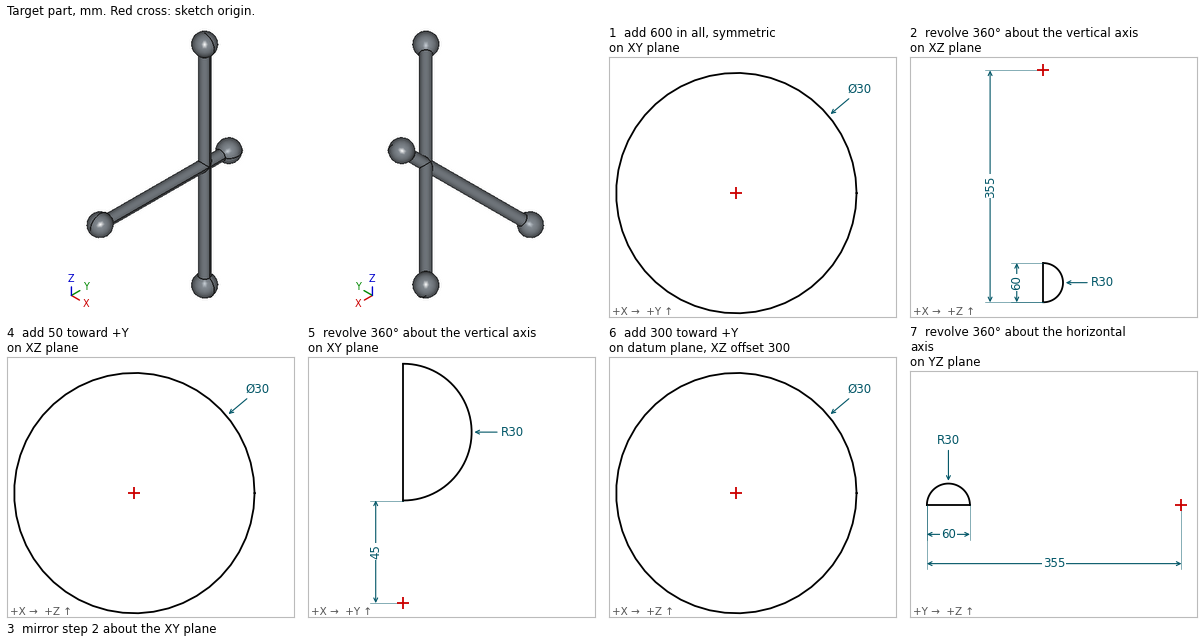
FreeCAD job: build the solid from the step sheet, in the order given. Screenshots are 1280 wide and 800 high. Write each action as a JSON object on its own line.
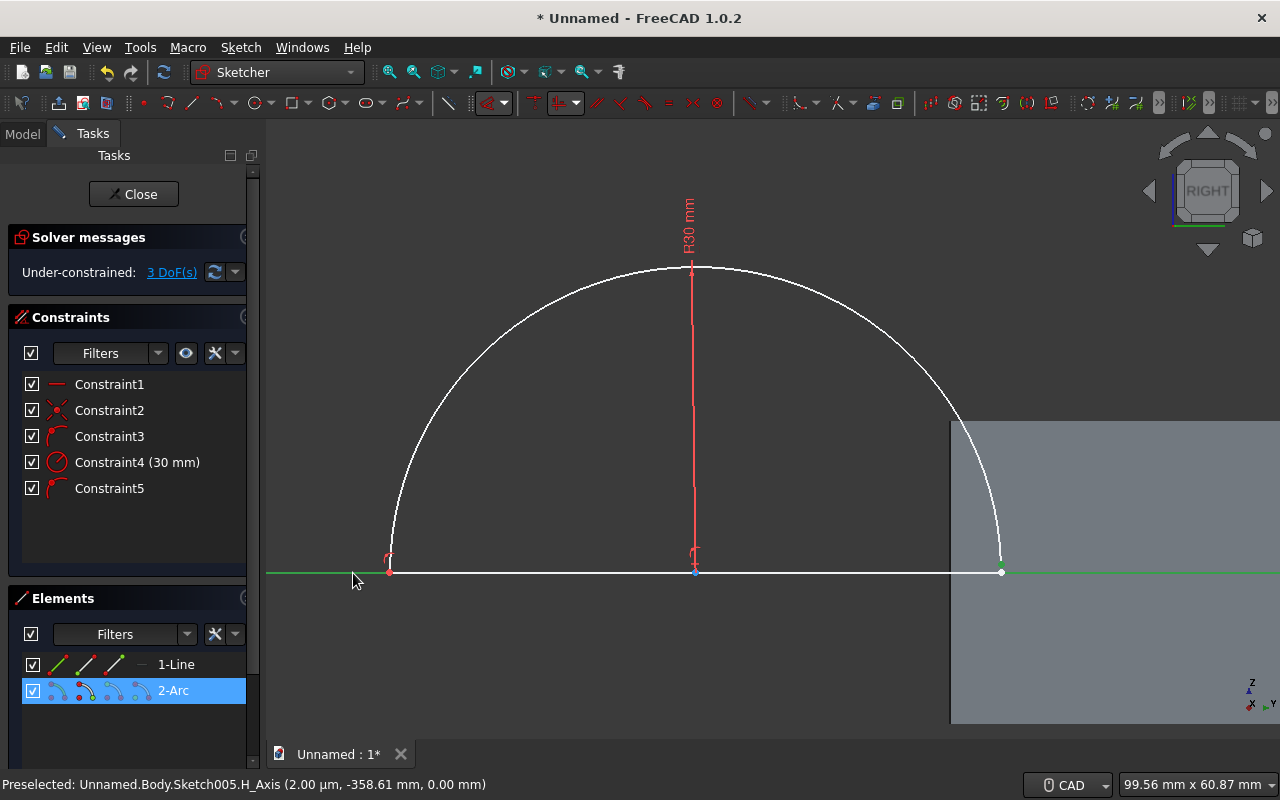
{"action": "left_click", "coordinate": [534, 104]}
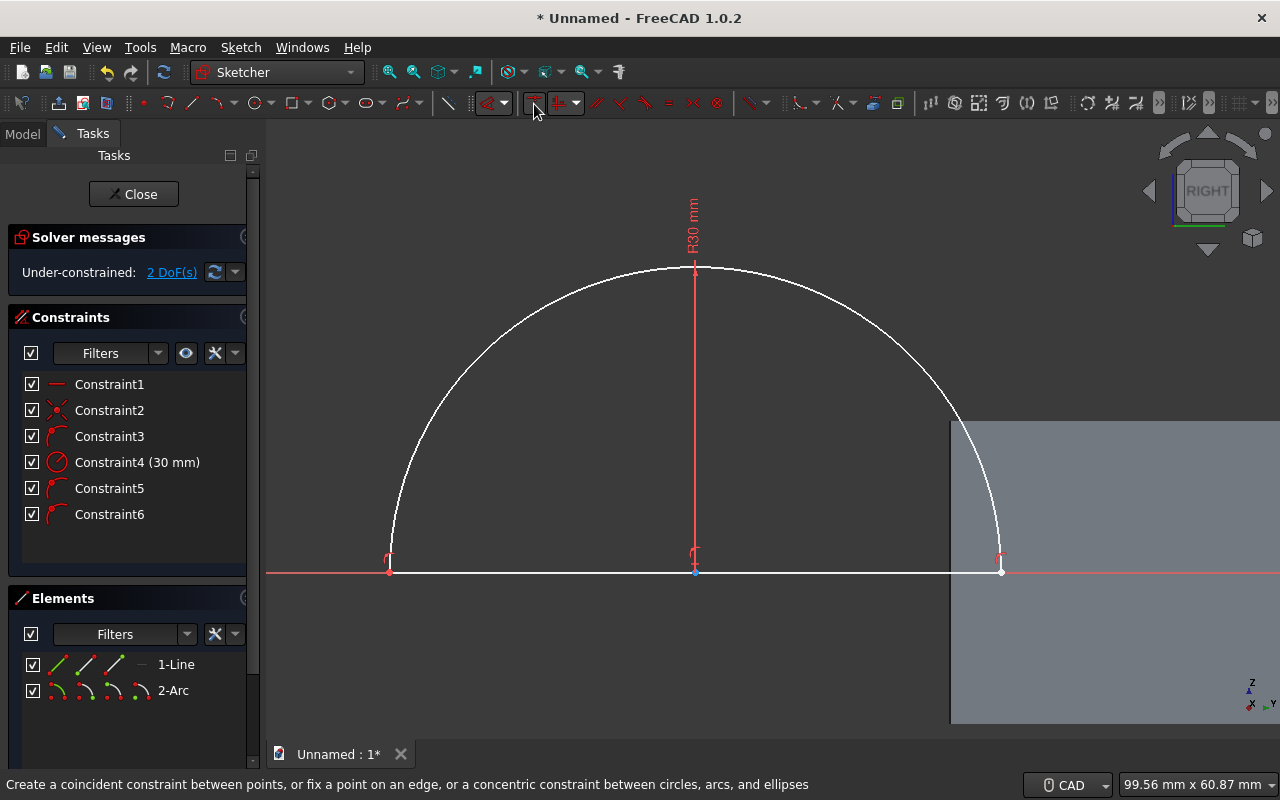
{"action": "left_click", "coordinate": [573, 573]}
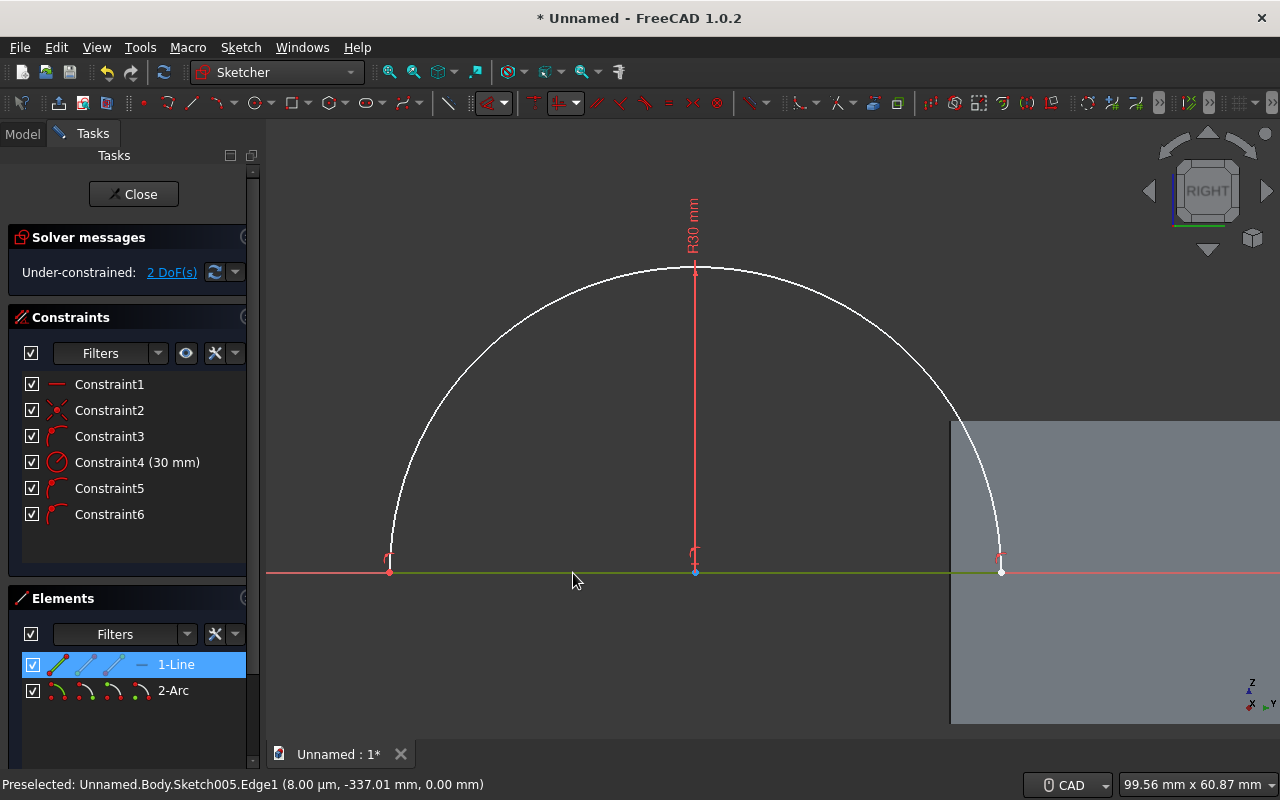
{"action": "key", "text": "l"}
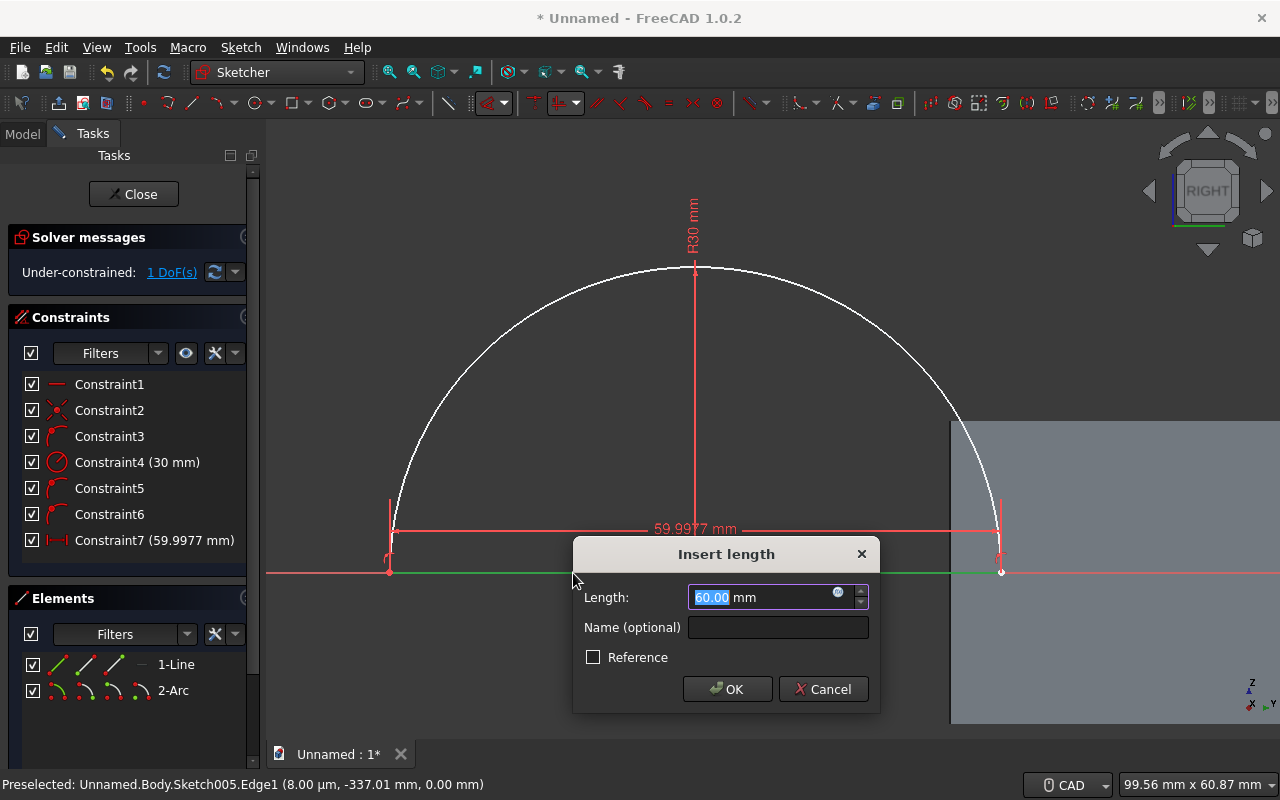
{"action": "type", "text": "60"}
{"action": "key", "text": "Return"}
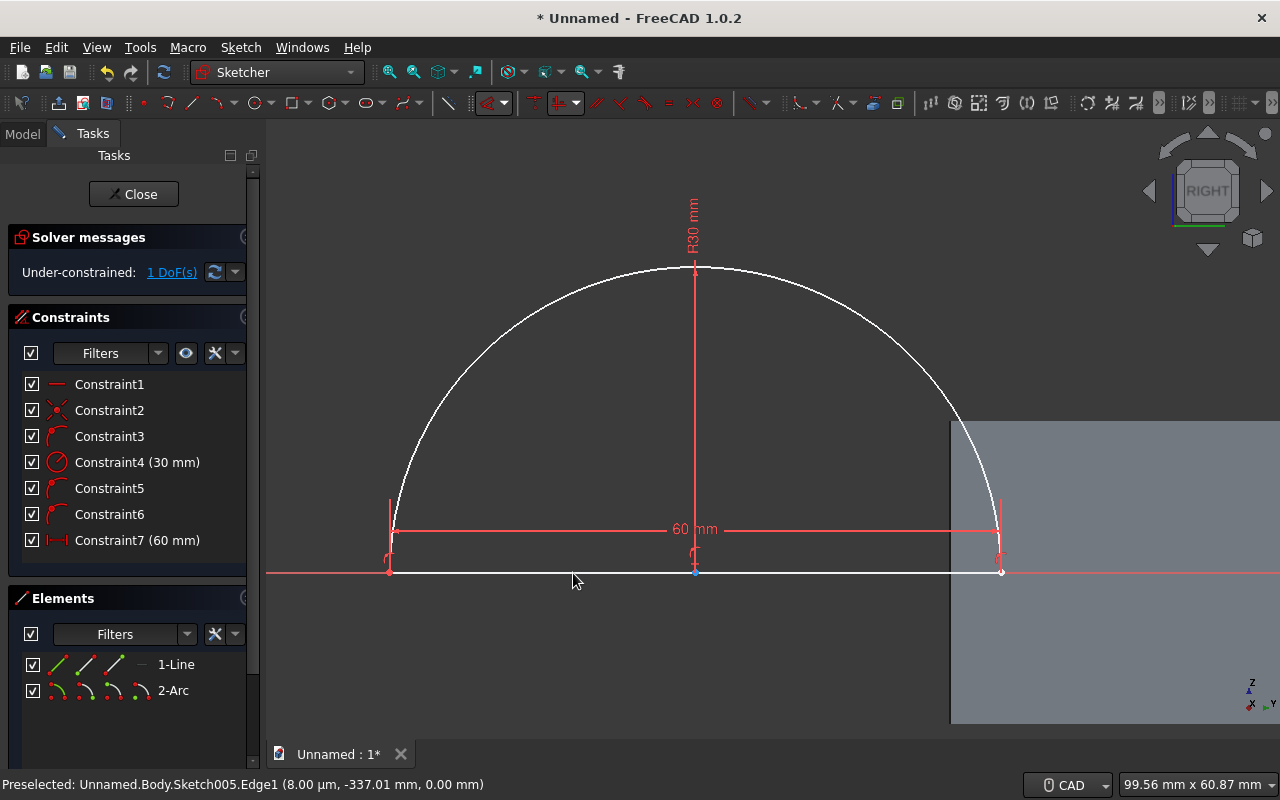
{"action": "left_click", "coordinate": [390, 573]}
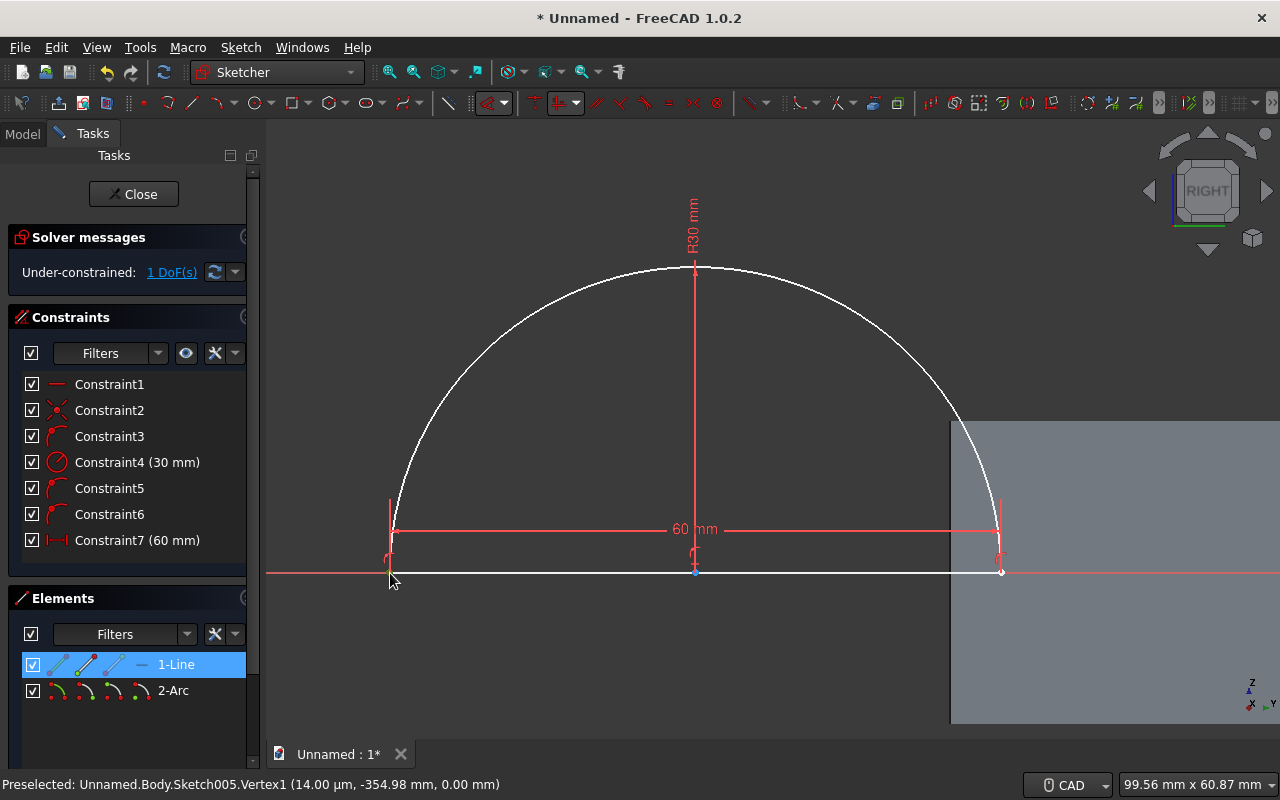
{"action": "key", "text": "l"}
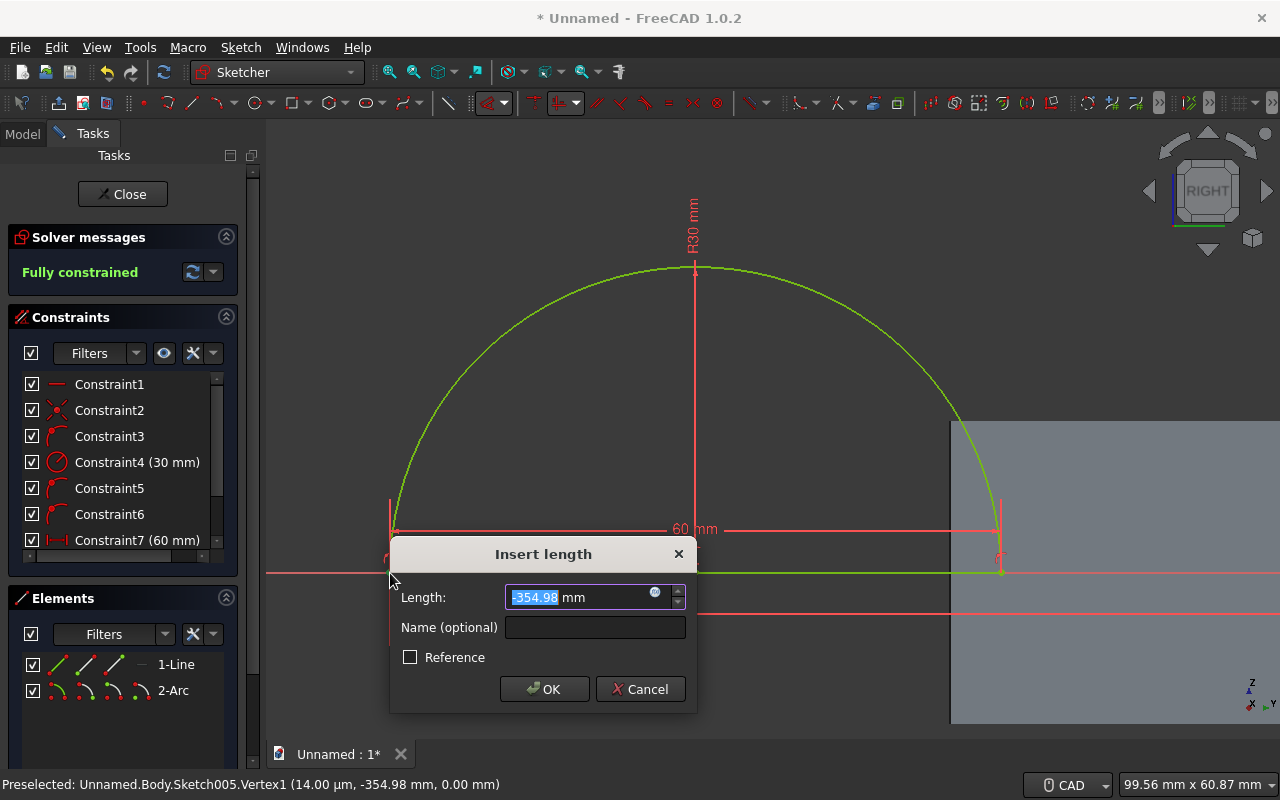
{"action": "type", "text": "-355"}
{"action": "key", "text": "Return"}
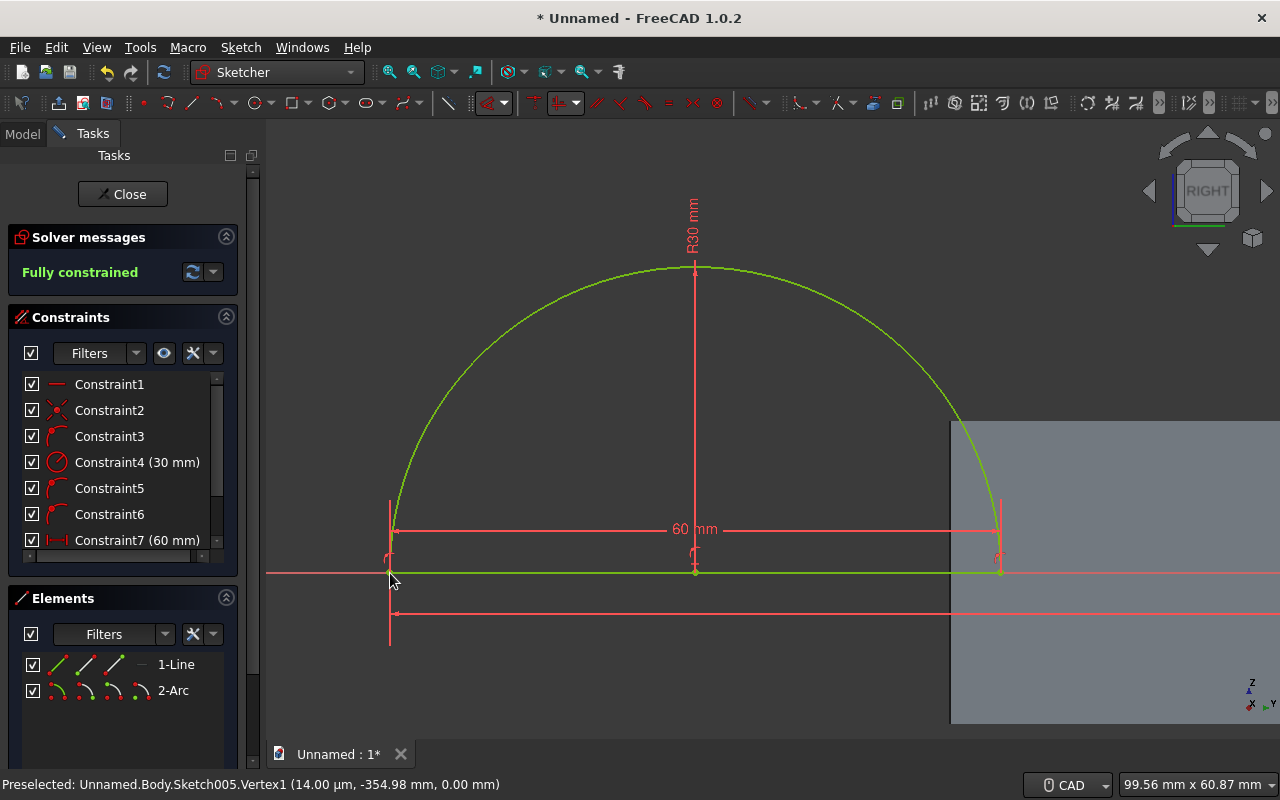
{"action": "left_click", "coordinate": [123, 194]}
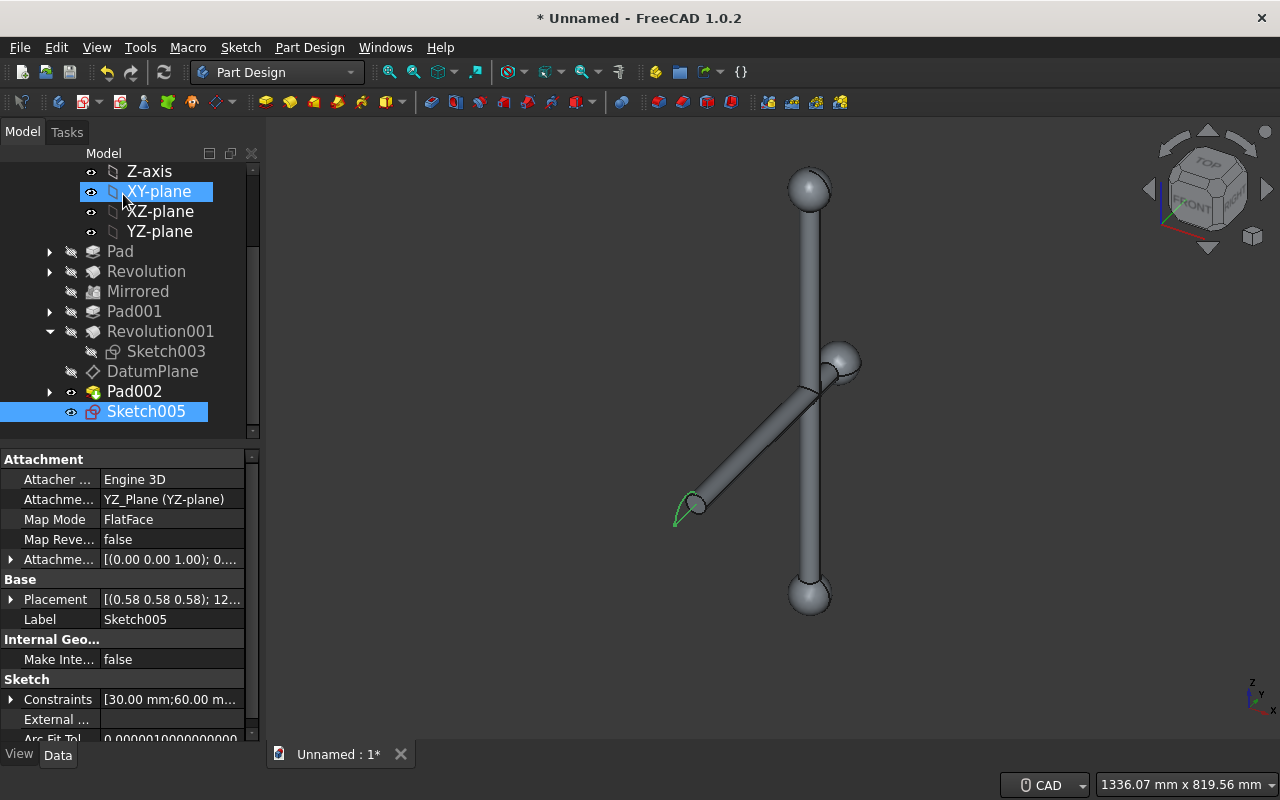
{"action": "left_click", "coordinate": [290, 102]}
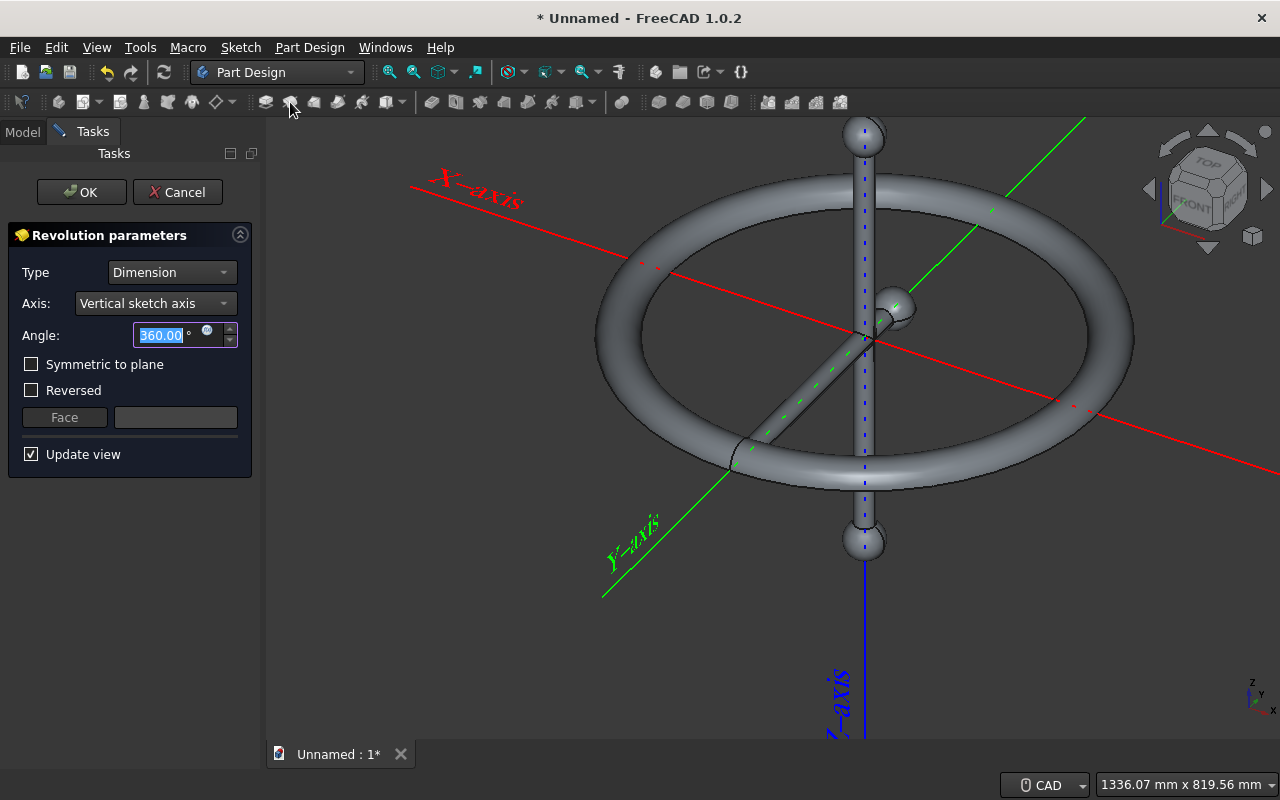
{"action": "left_click", "coordinate": [156, 304]}